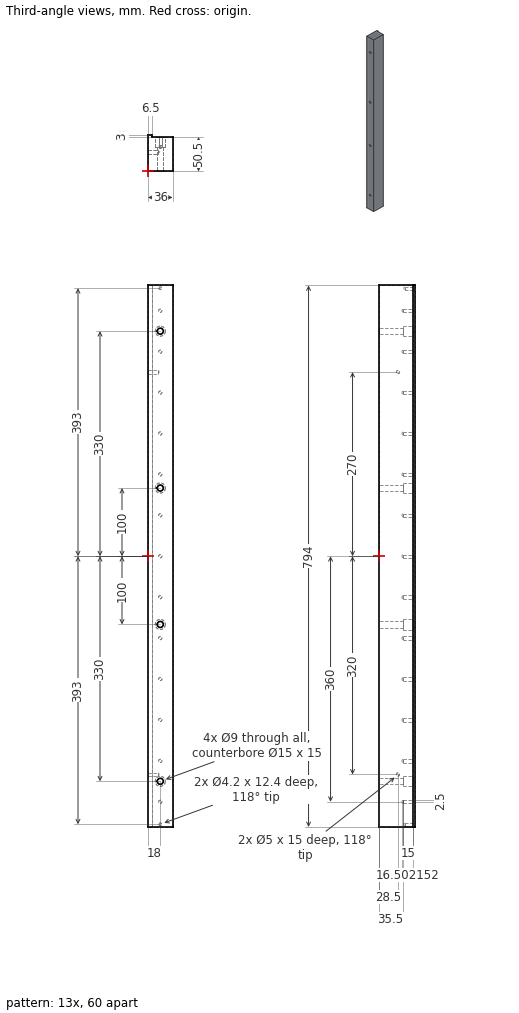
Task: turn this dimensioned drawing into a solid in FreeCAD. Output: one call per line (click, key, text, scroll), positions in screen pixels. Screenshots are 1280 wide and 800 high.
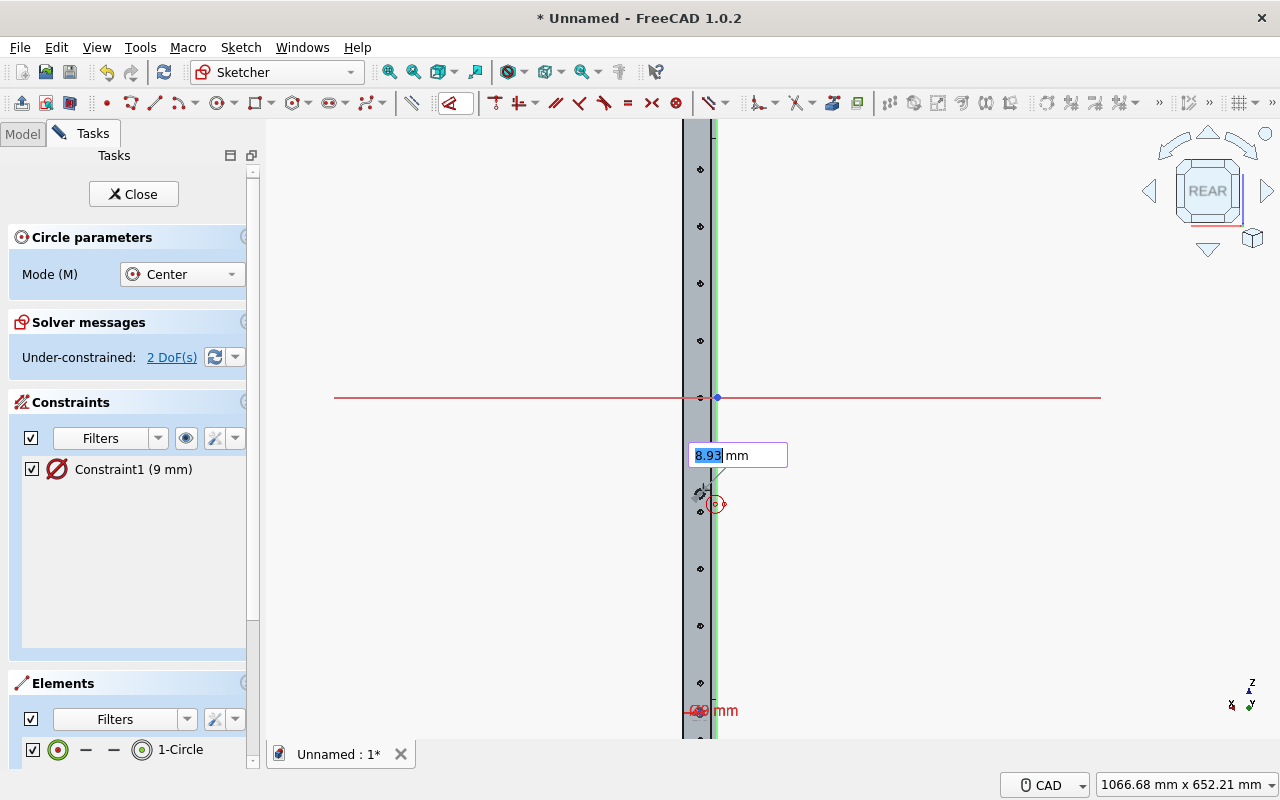
text(9)
key(Return)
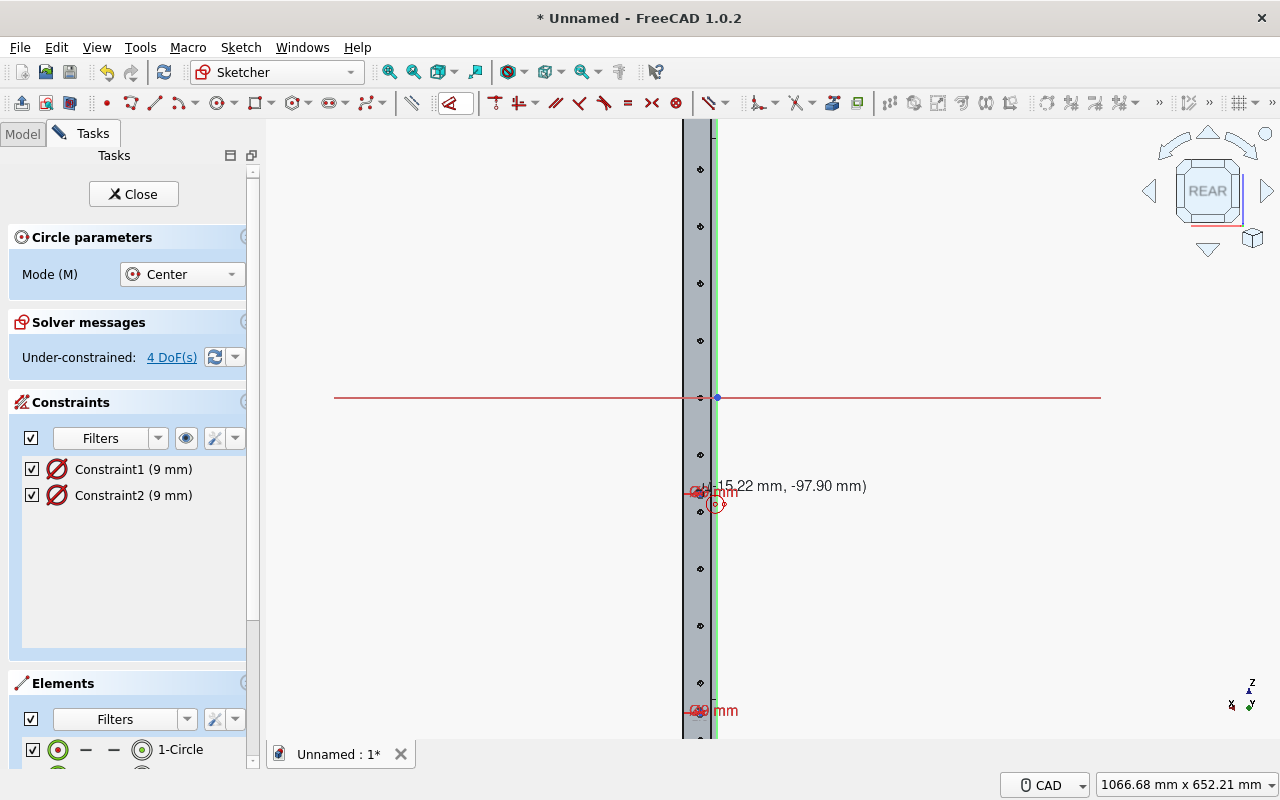
scroll(700, 303, up, 9)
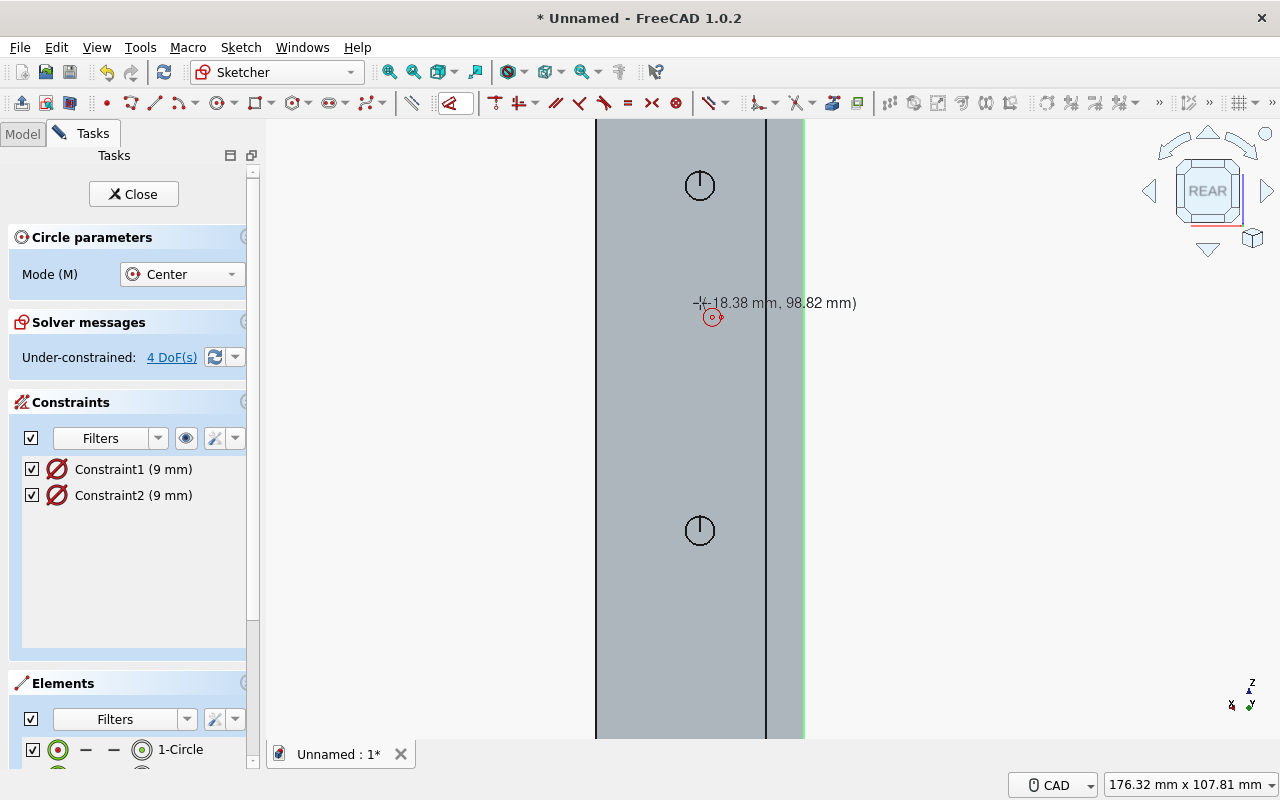
scroll(700, 373, down, 11)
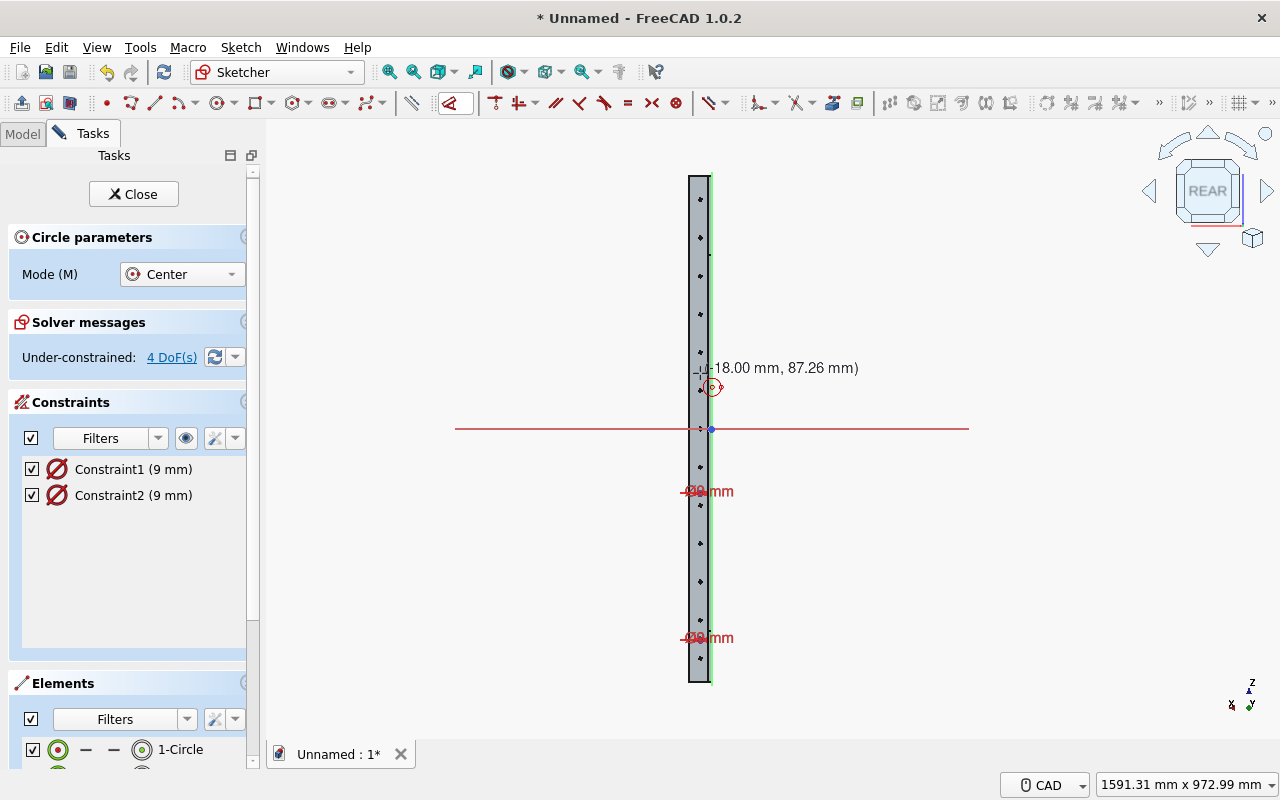
scroll(700, 365, up, 2)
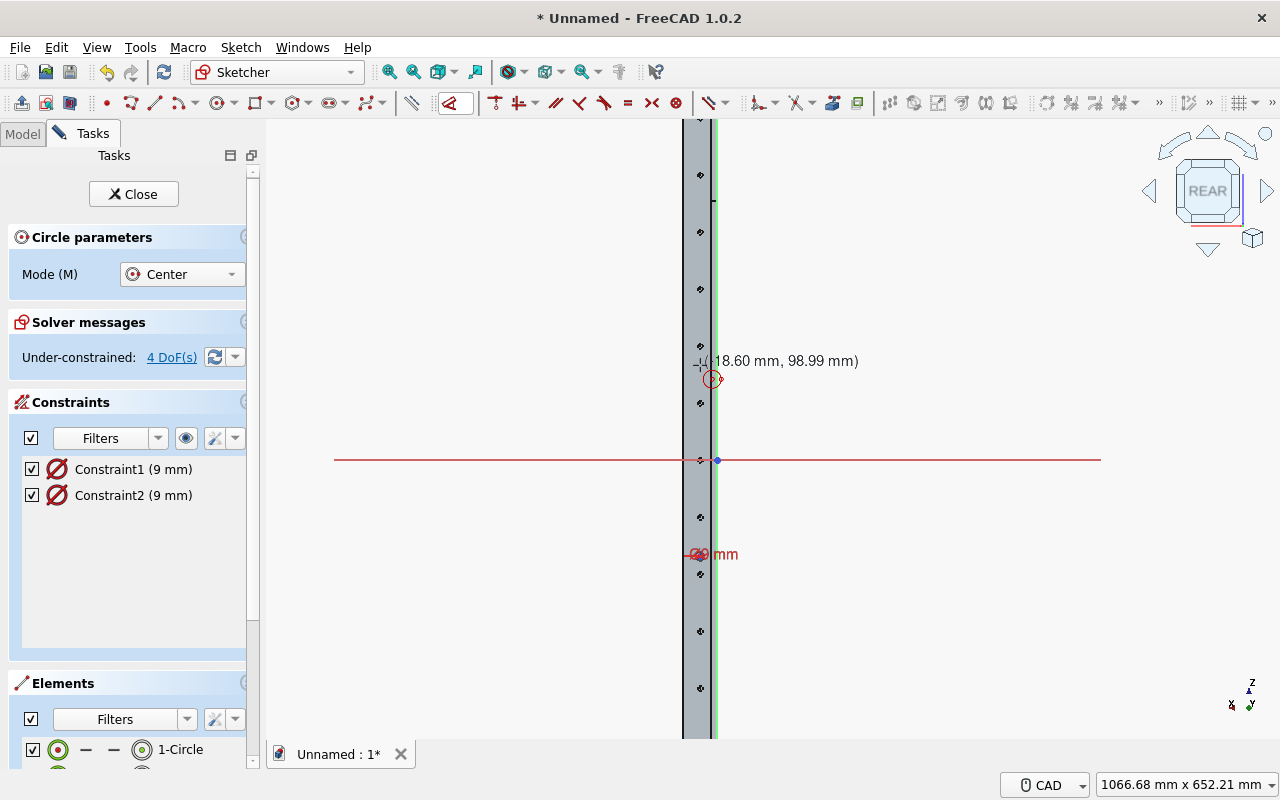
click(700, 365)
move(703, 362)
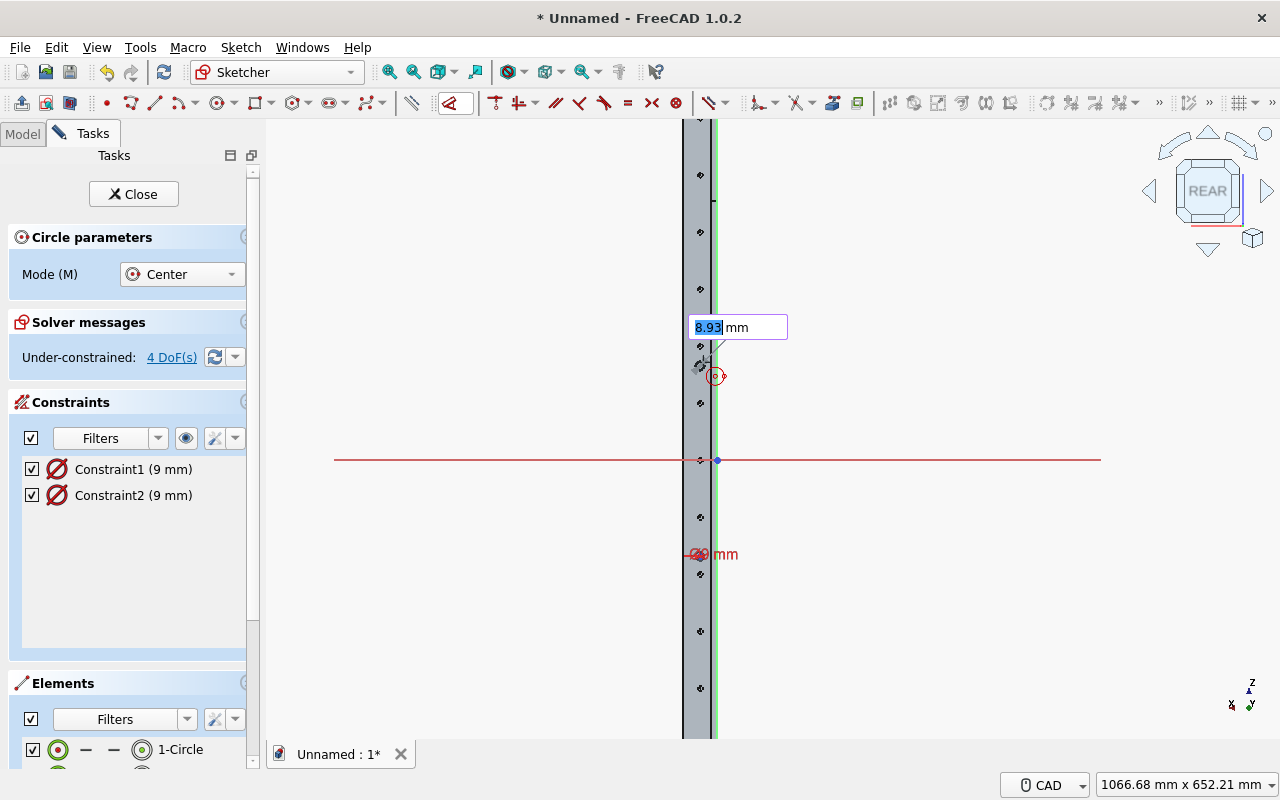
text(9)
key(Return)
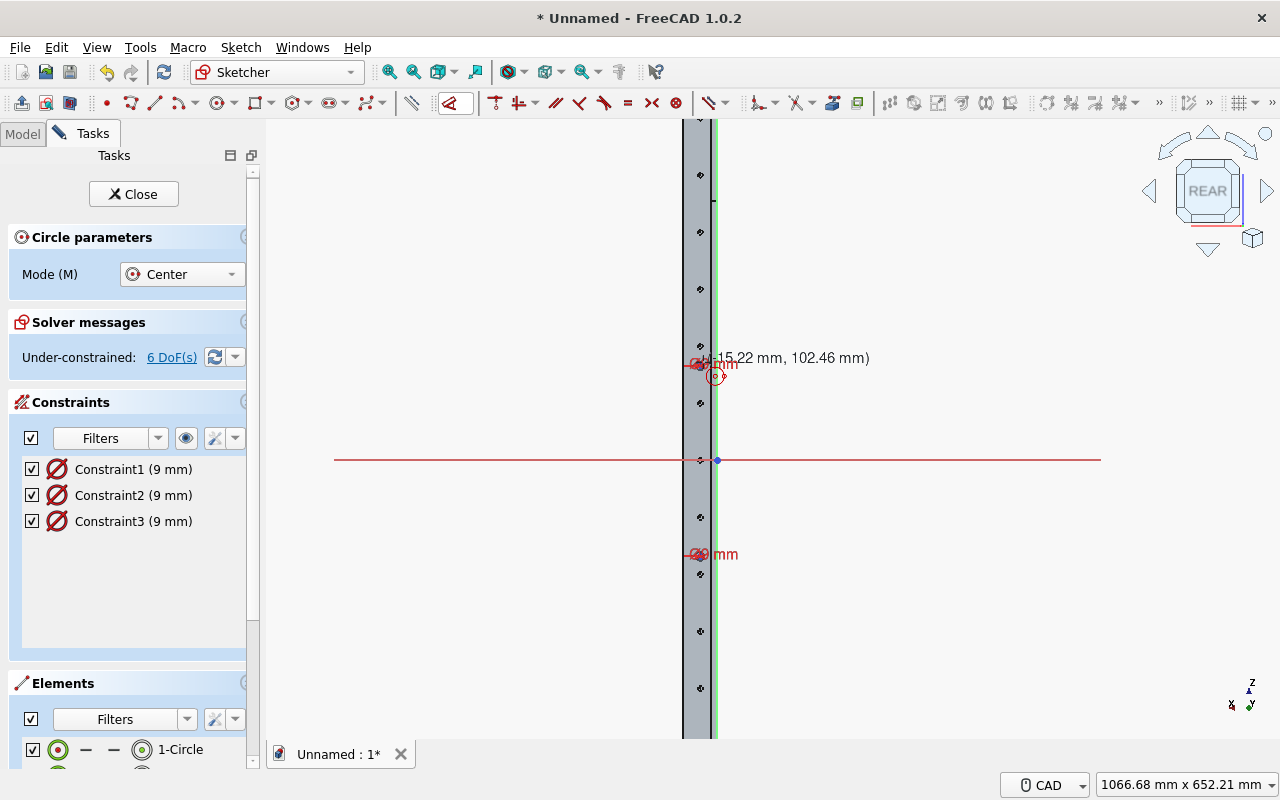
scroll(700, 365, down, 2)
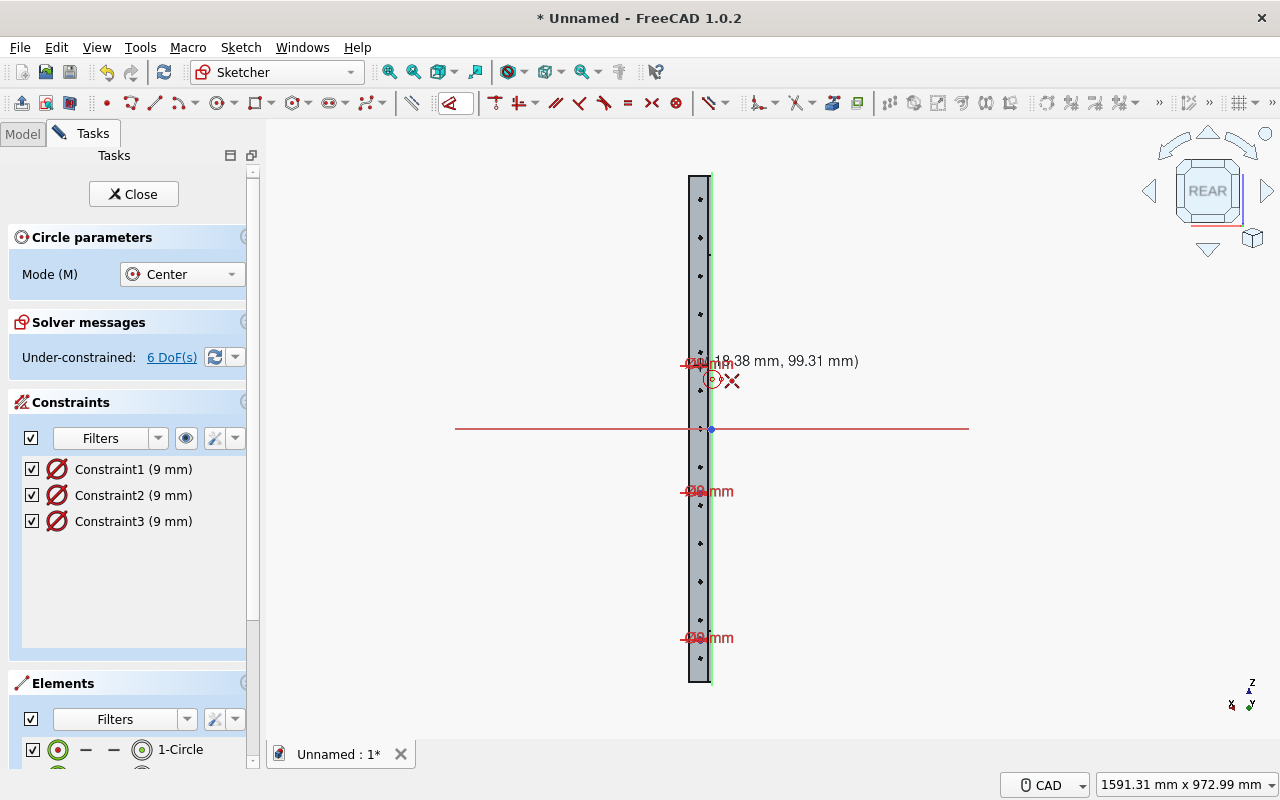
scroll(700, 219, up, 11)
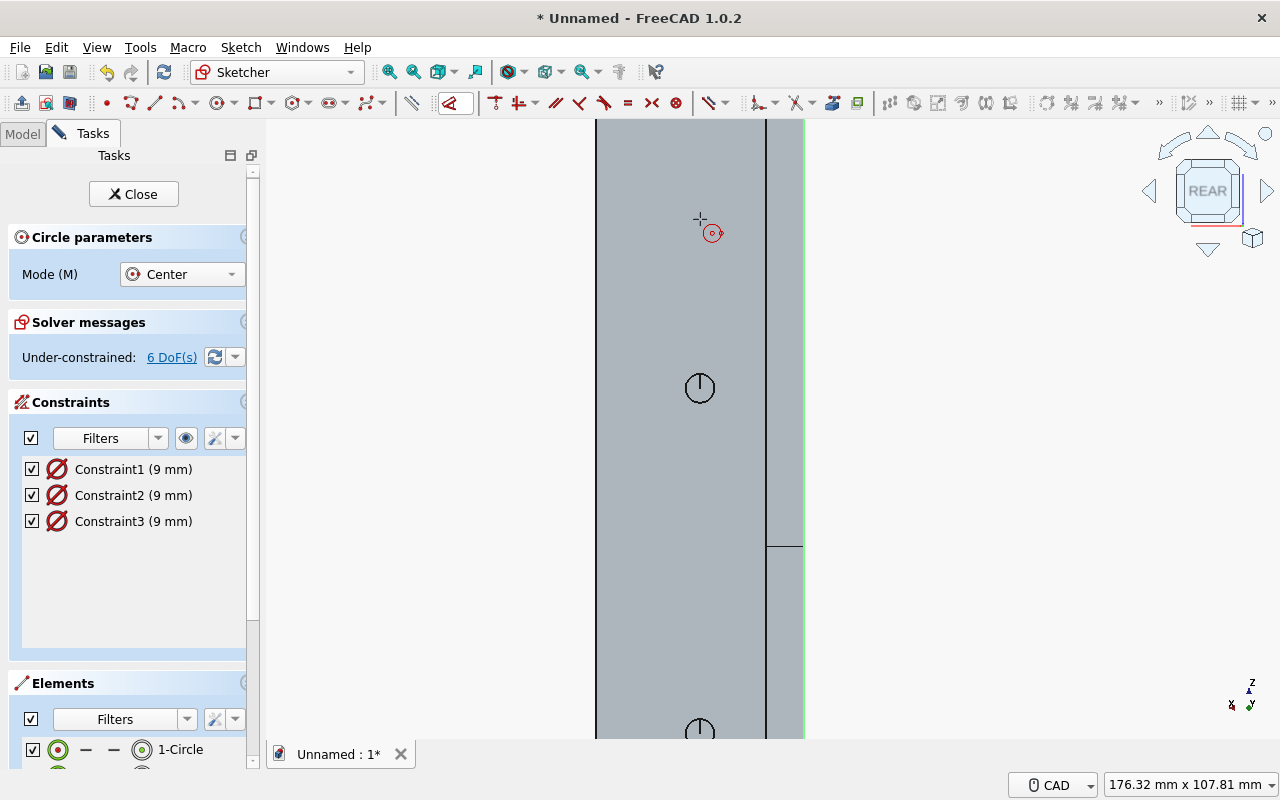
scroll(700, 219, down, 11)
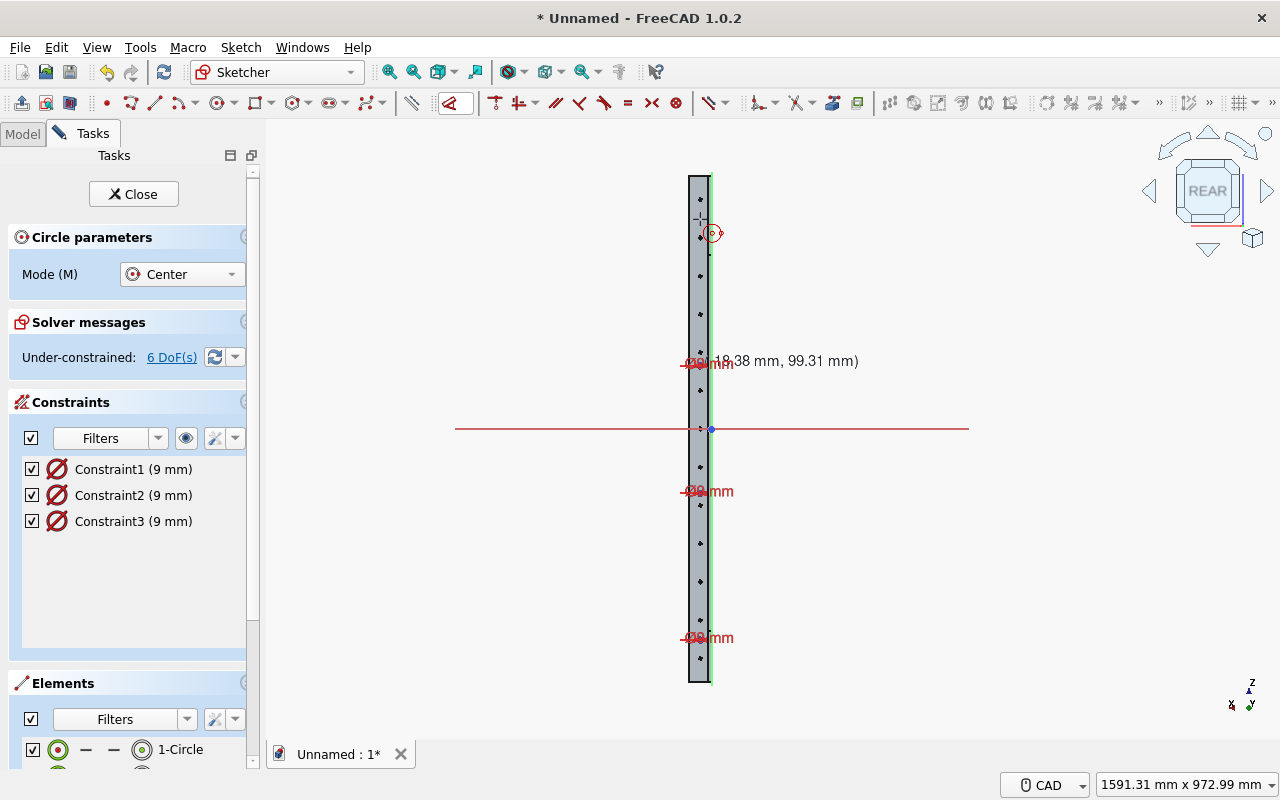
scroll(700, 219, up, 2)